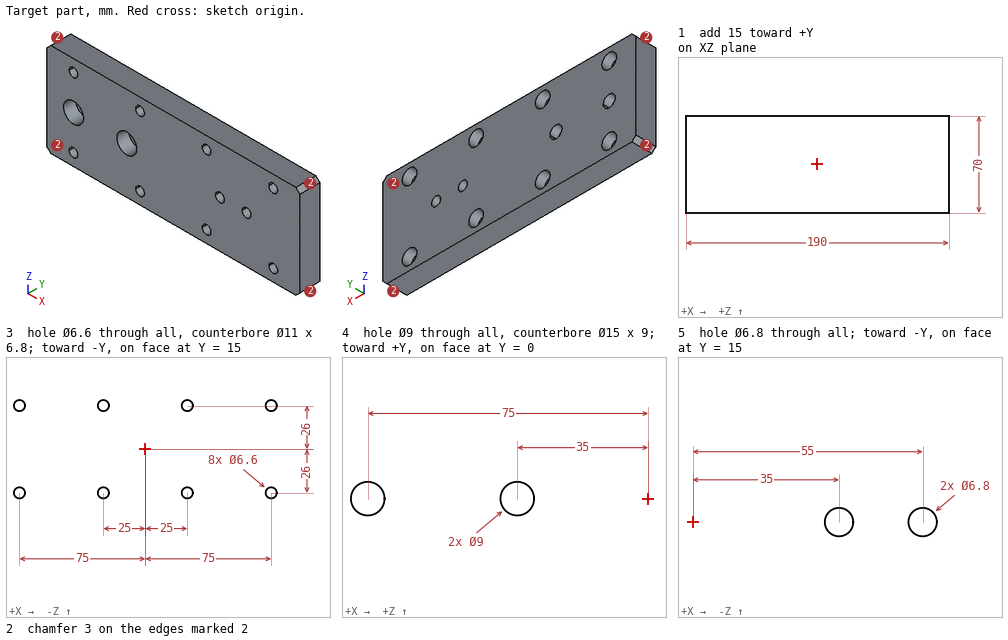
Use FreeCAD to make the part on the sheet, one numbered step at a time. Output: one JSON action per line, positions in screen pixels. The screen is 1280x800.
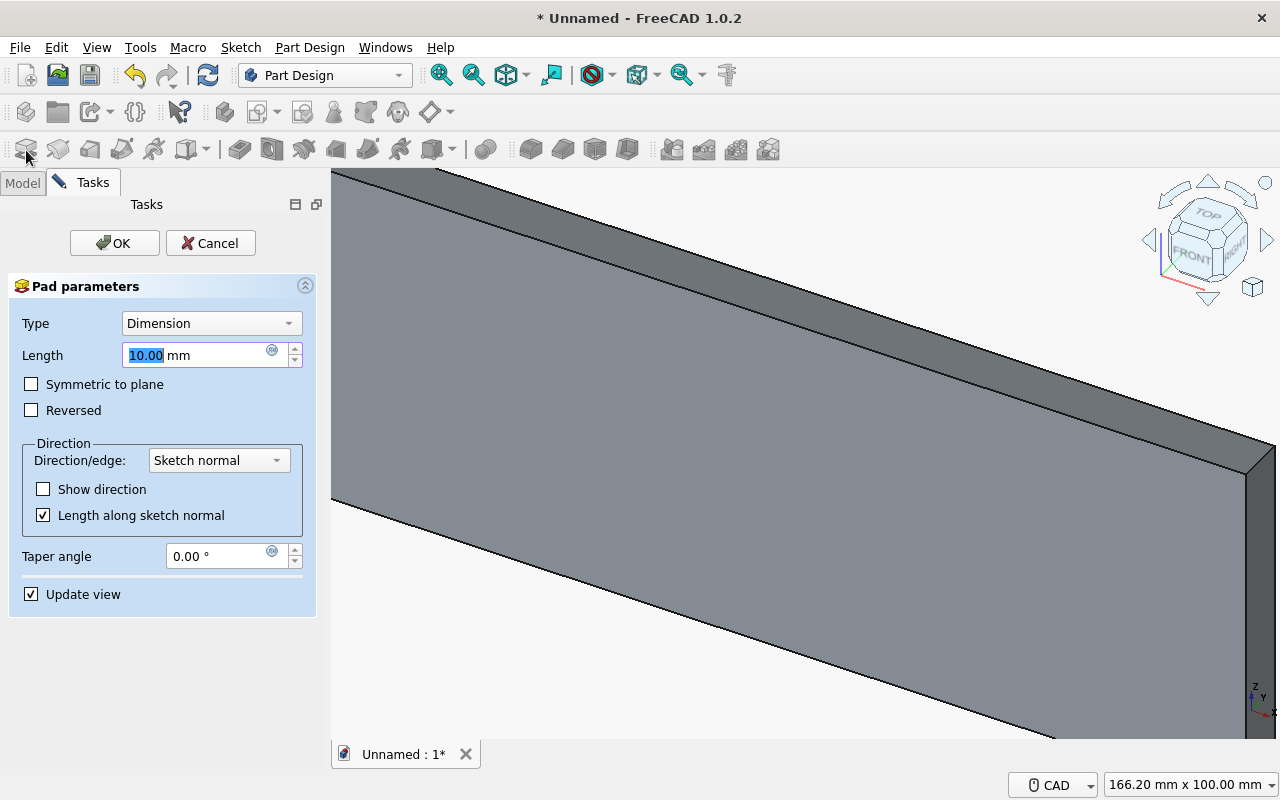
{"action": "type", "text": "15"}
{"action": "key", "text": "Tab"}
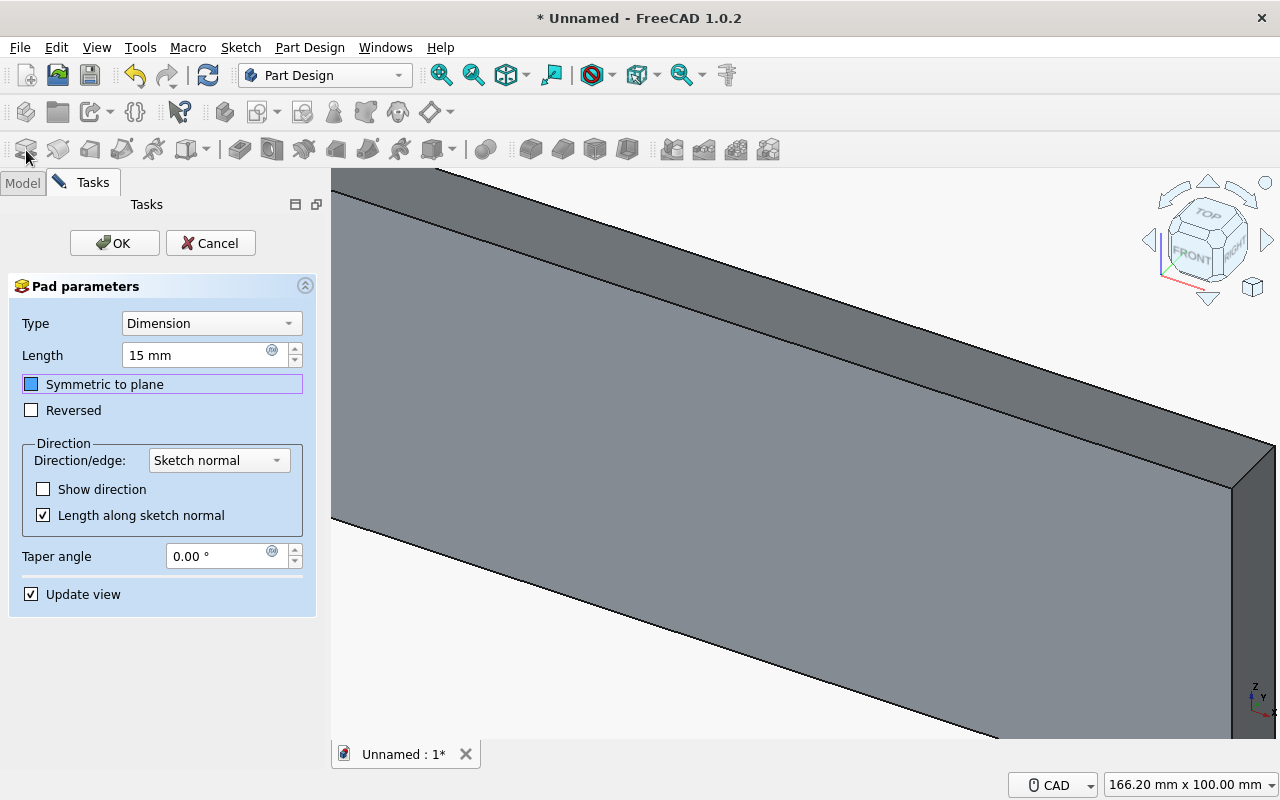
{"action": "left_click", "coordinate": [30, 410]}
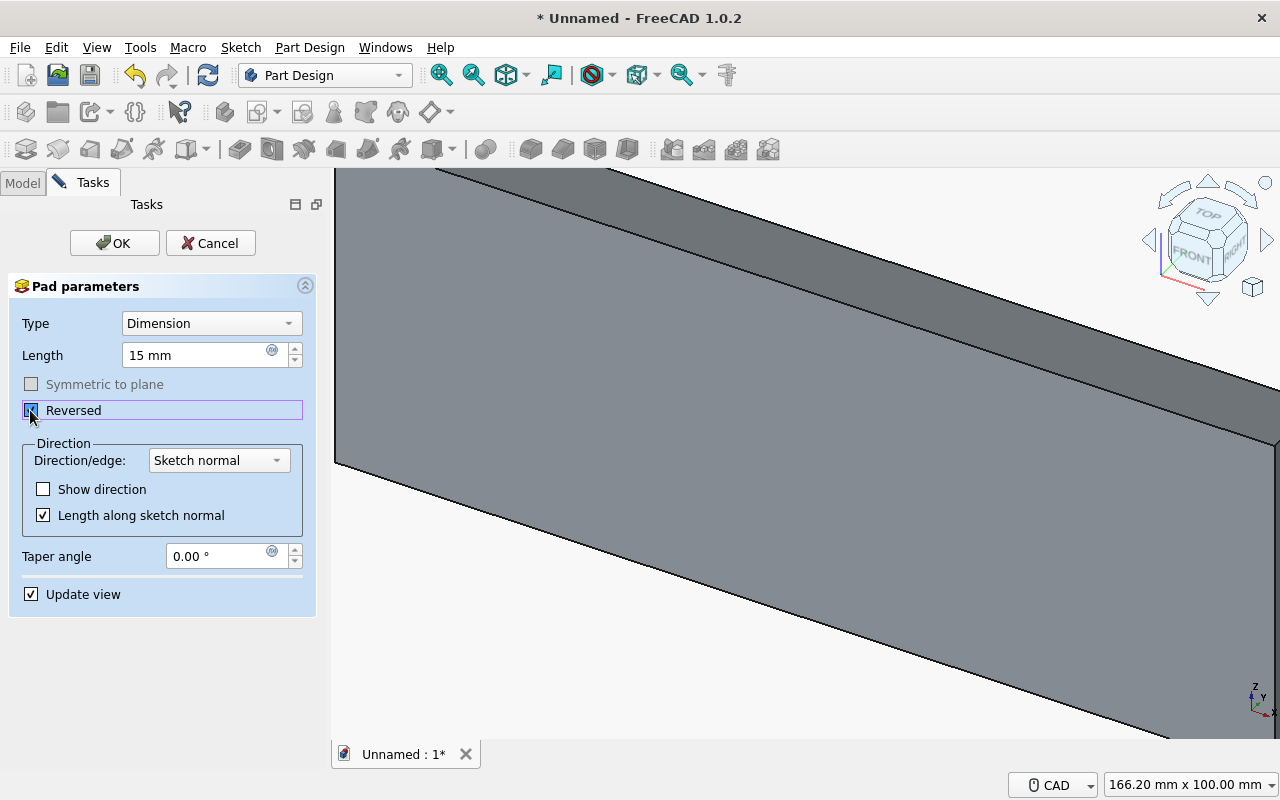
{"action": "left_click", "coordinate": [115, 243]}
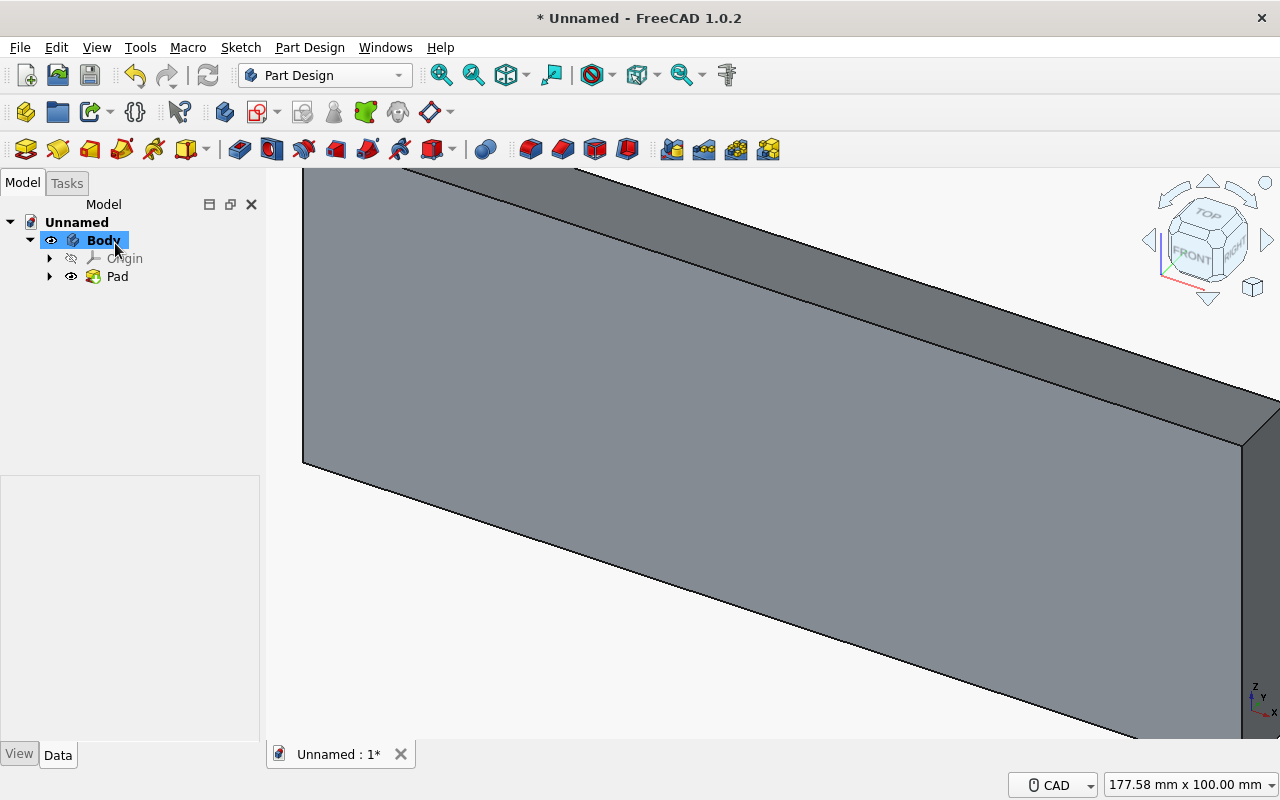
{"action": "key", "text": "v f"}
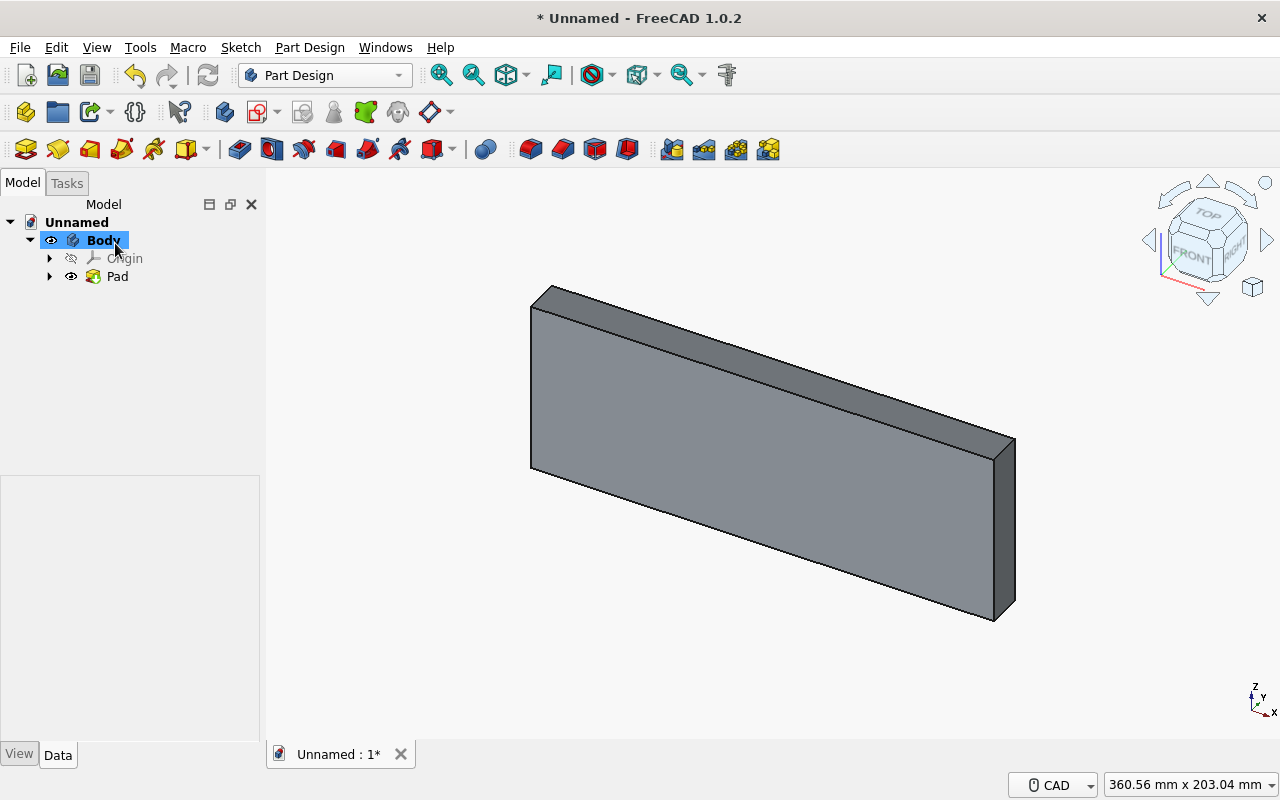
{"action": "left_click", "coordinate": [1004, 448]}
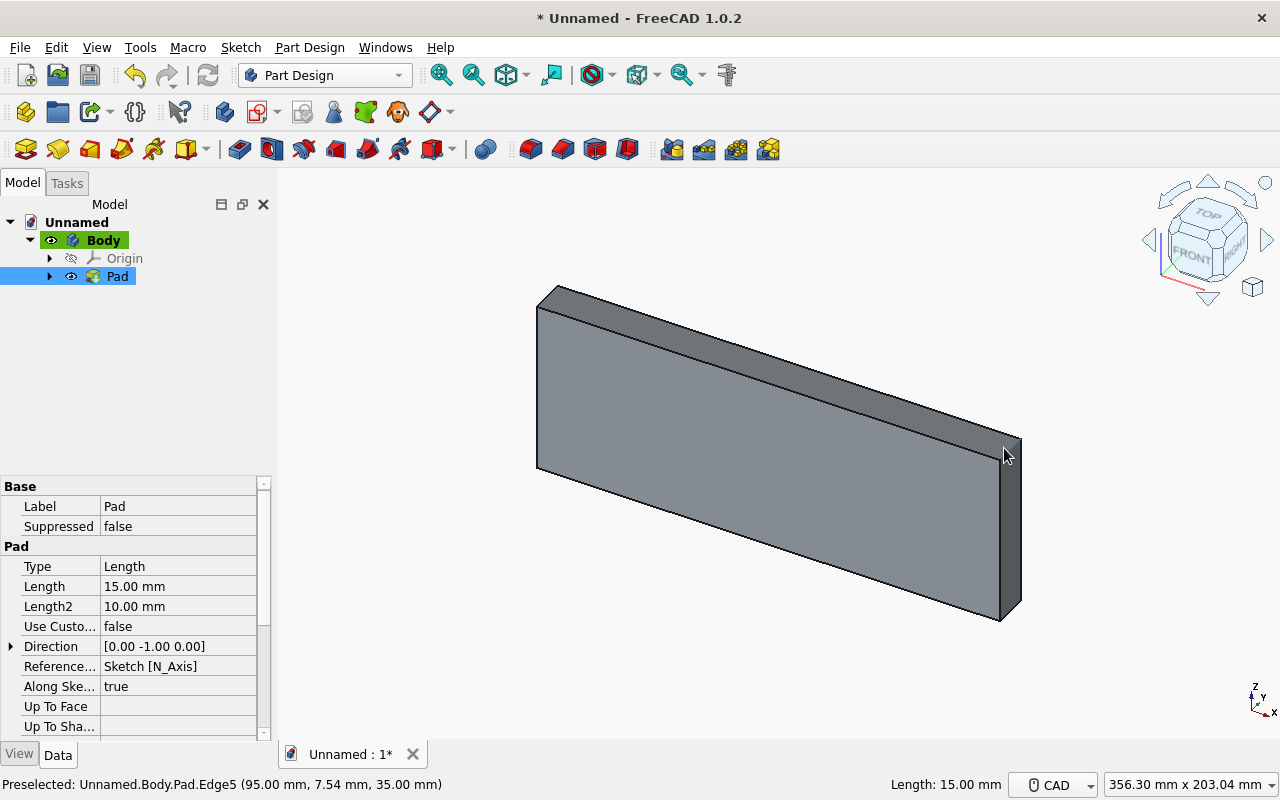
{"action": "key", "text": "0"}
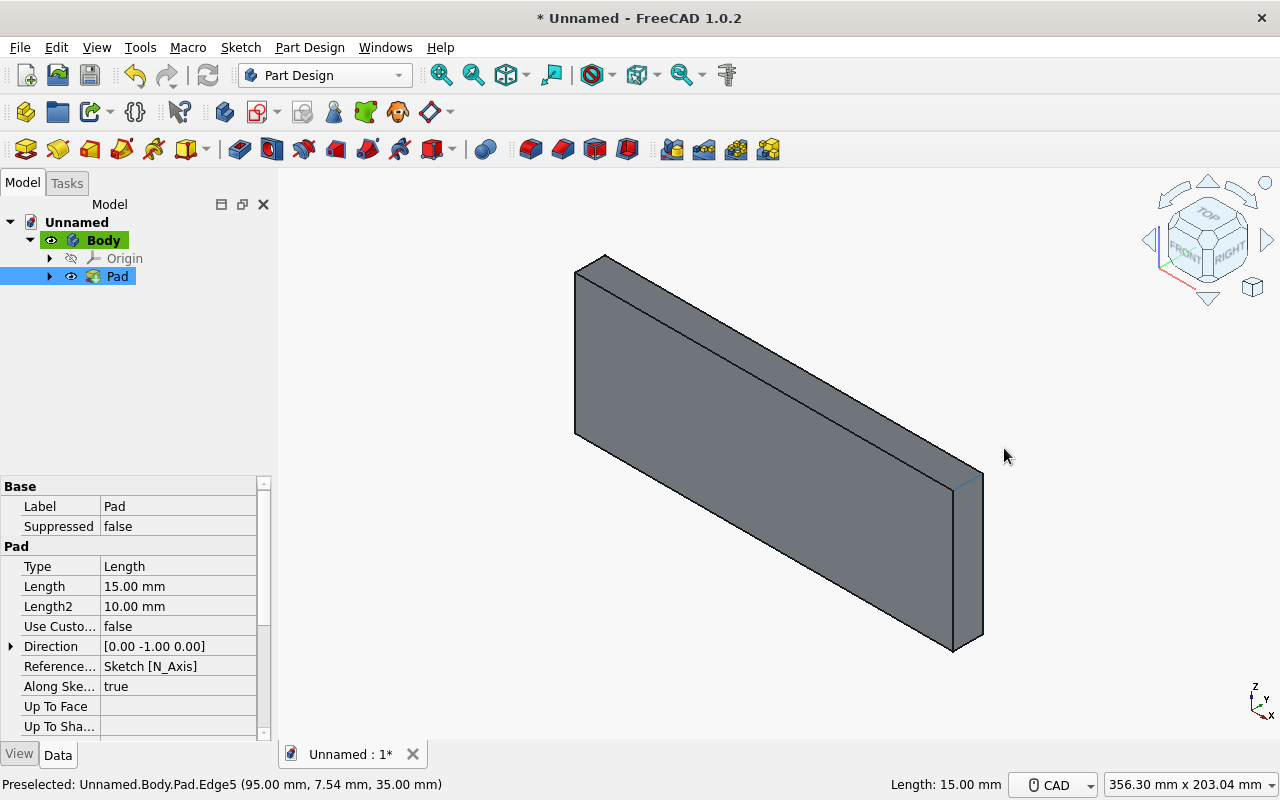
{"action": "key", "text": "2"}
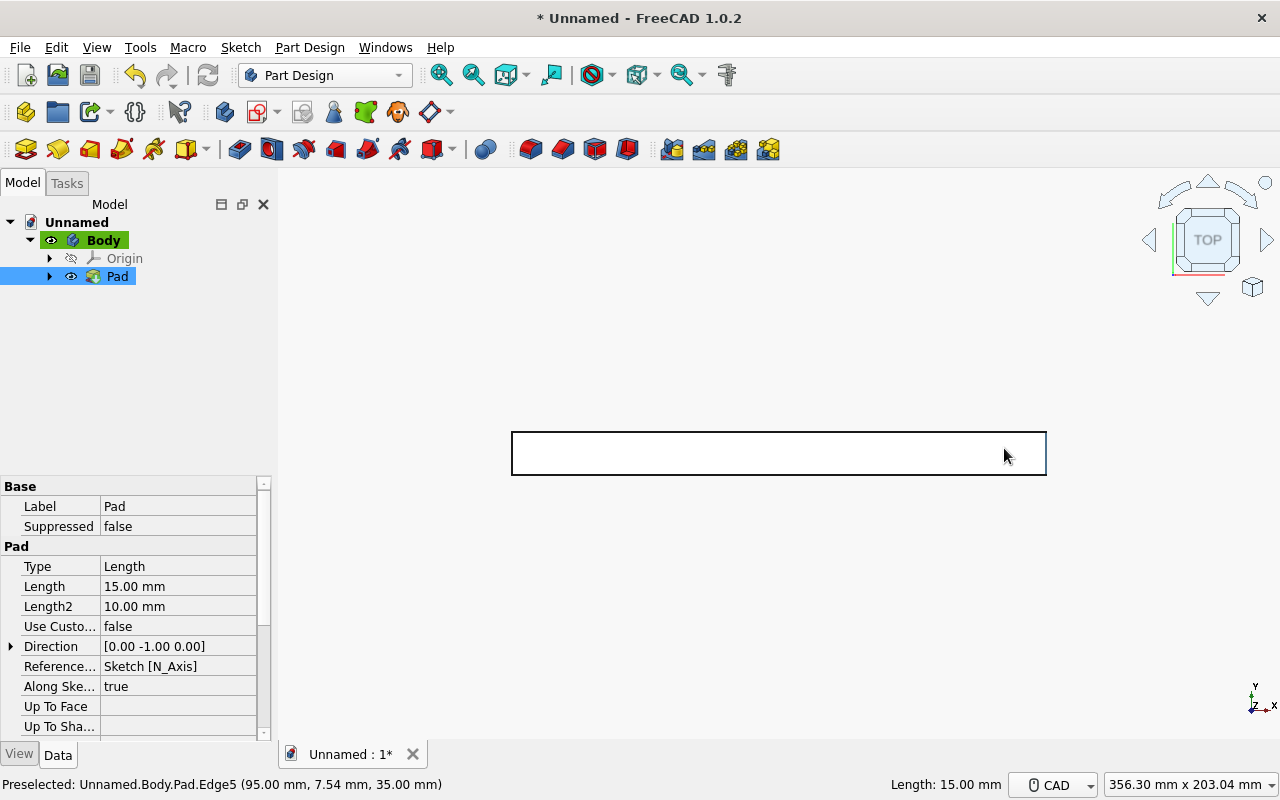
{"action": "left_click", "coordinate": [512, 452], "text": "ctrl"}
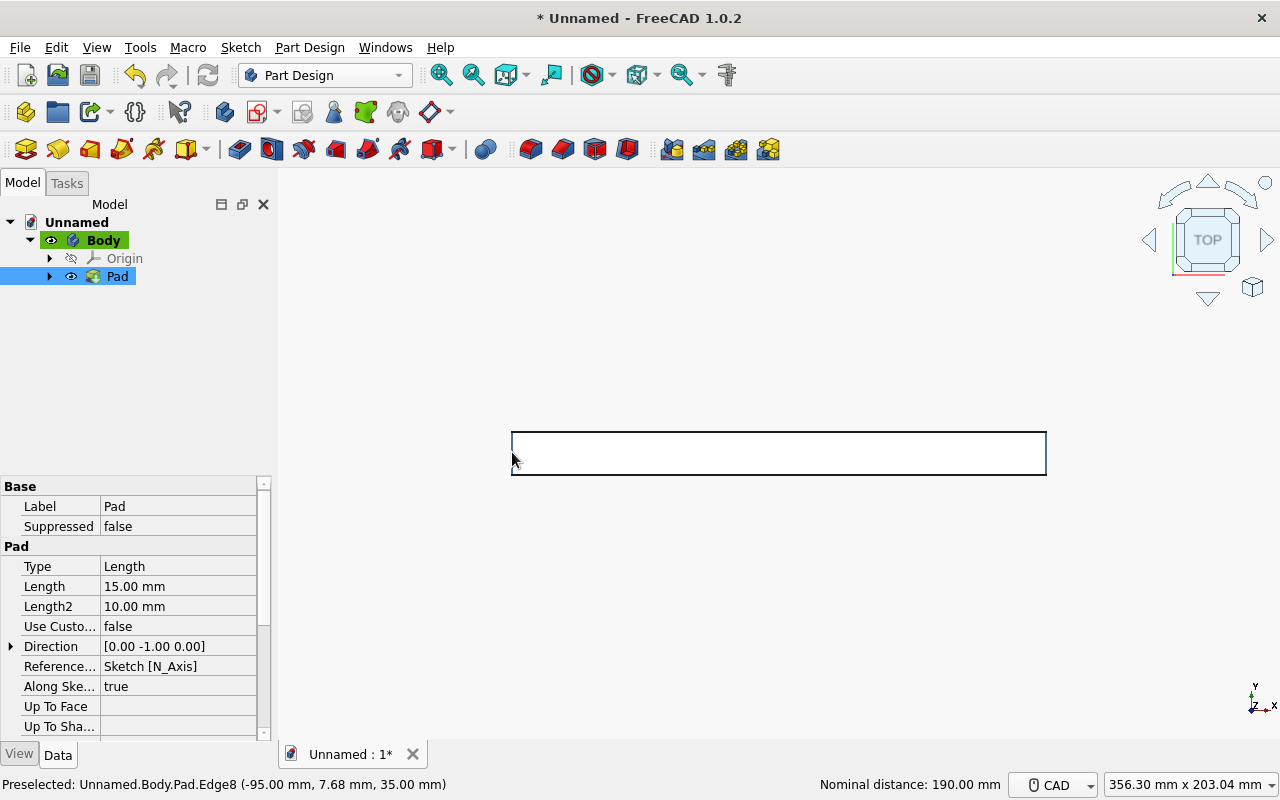
{"action": "key", "text": "1"}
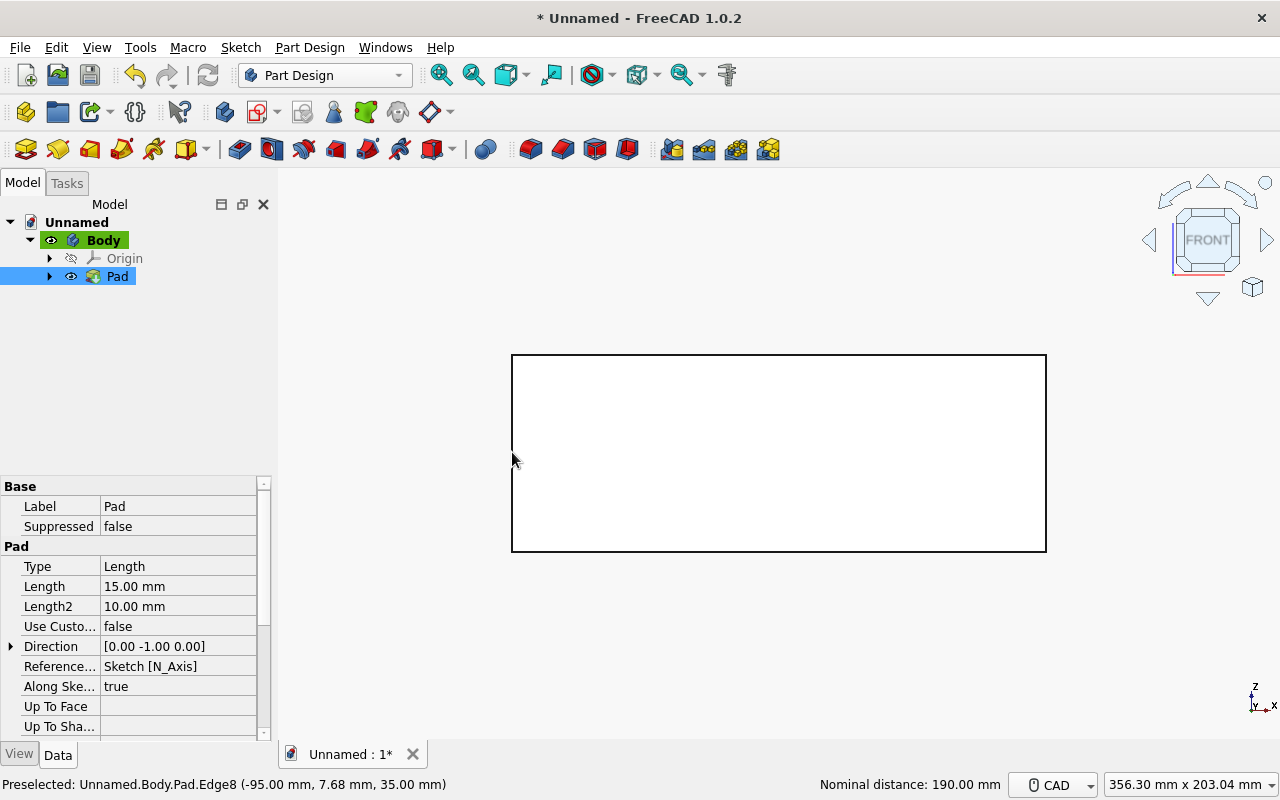
{"action": "key", "text": "3"}